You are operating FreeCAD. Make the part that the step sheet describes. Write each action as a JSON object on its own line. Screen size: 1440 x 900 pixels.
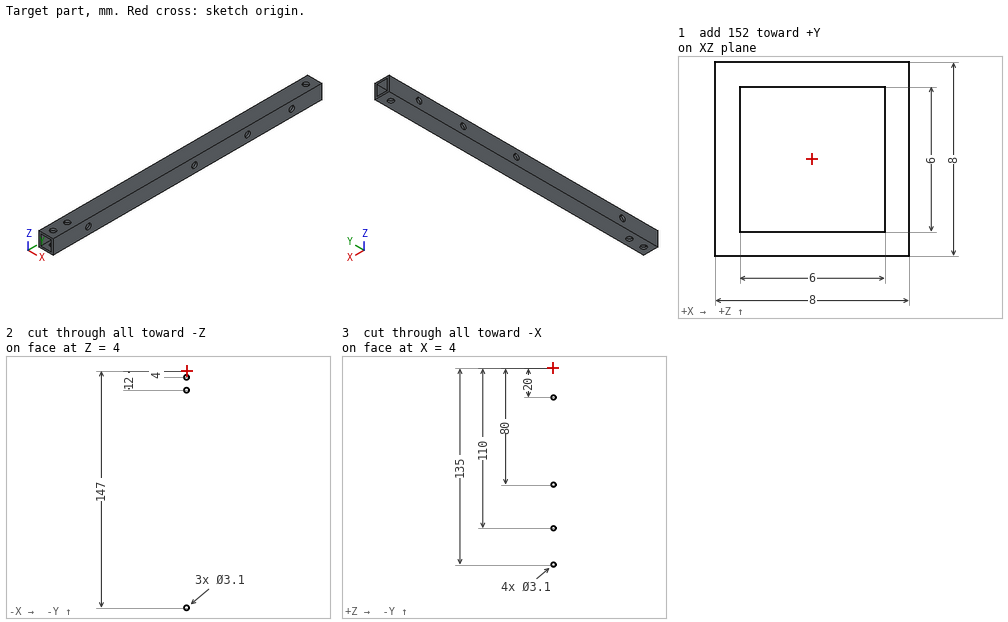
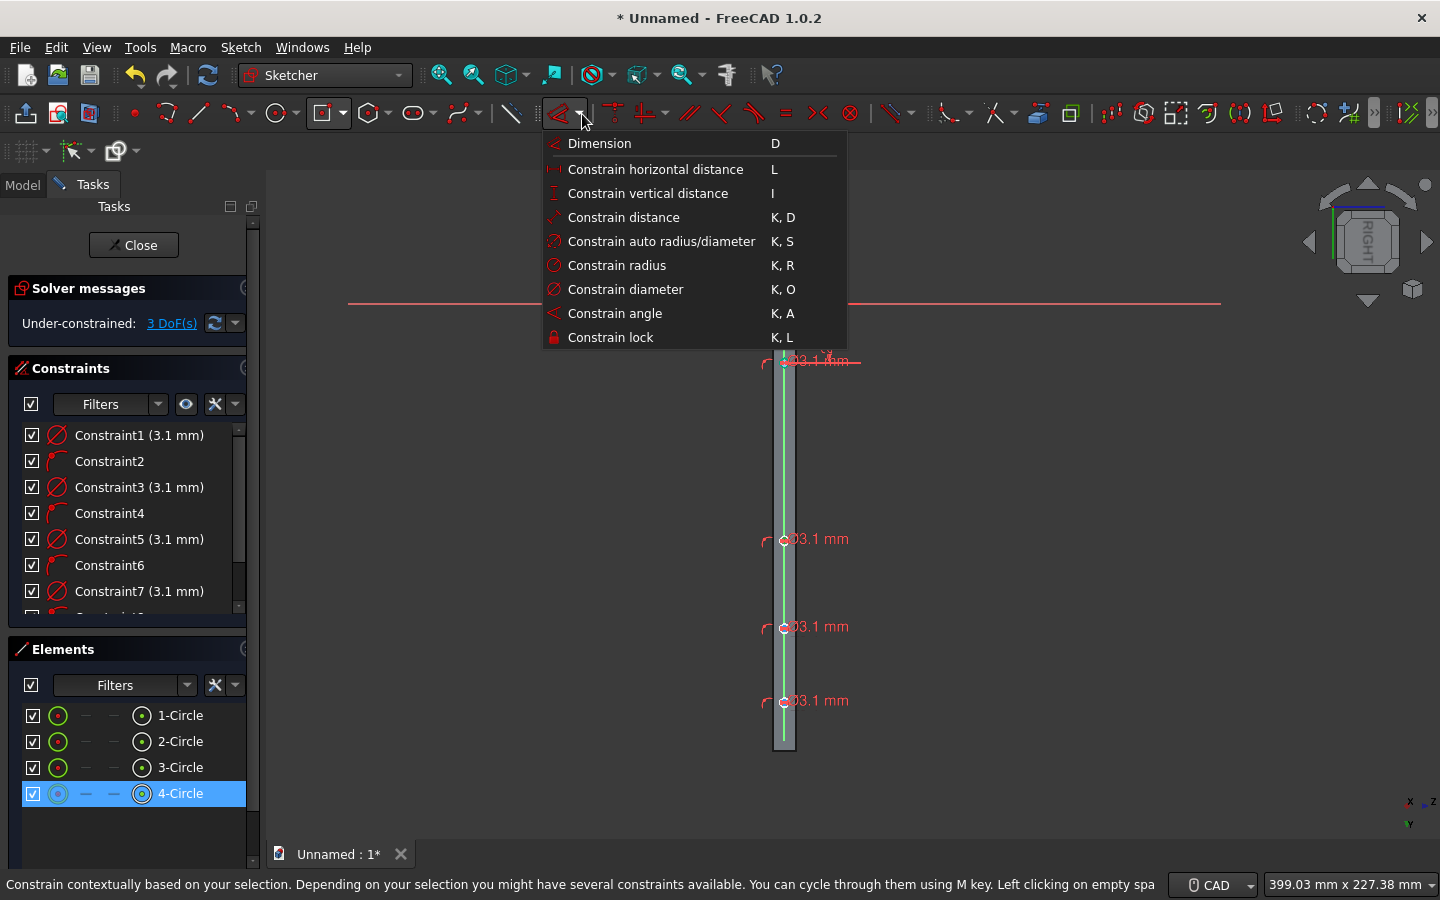
{"action": "left_click", "coordinate": [695, 193]}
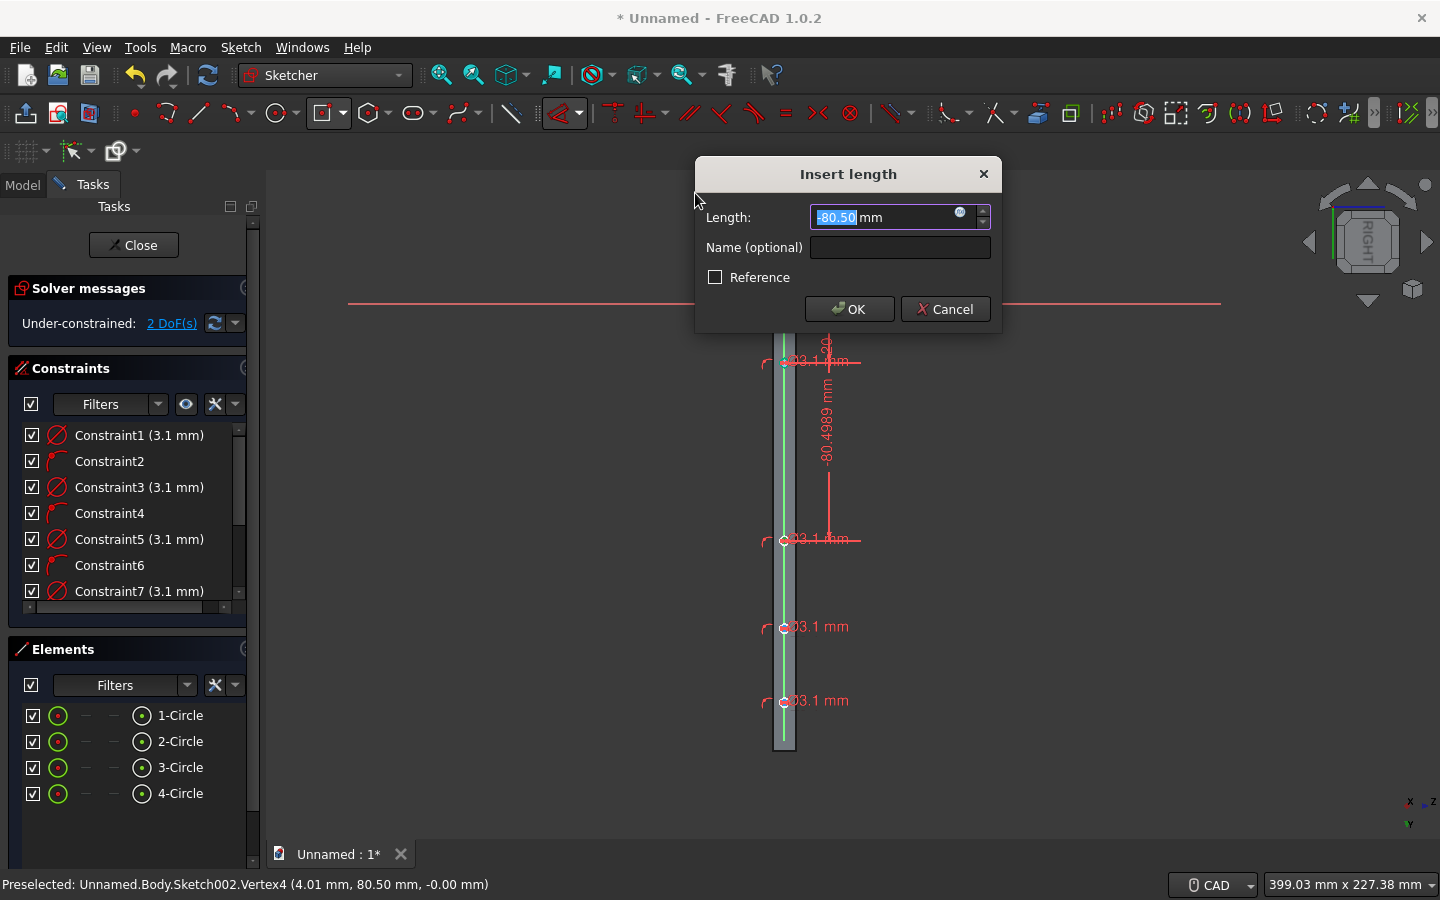
{"action": "type", "text": "-80"}
{"action": "key", "text": "Return"}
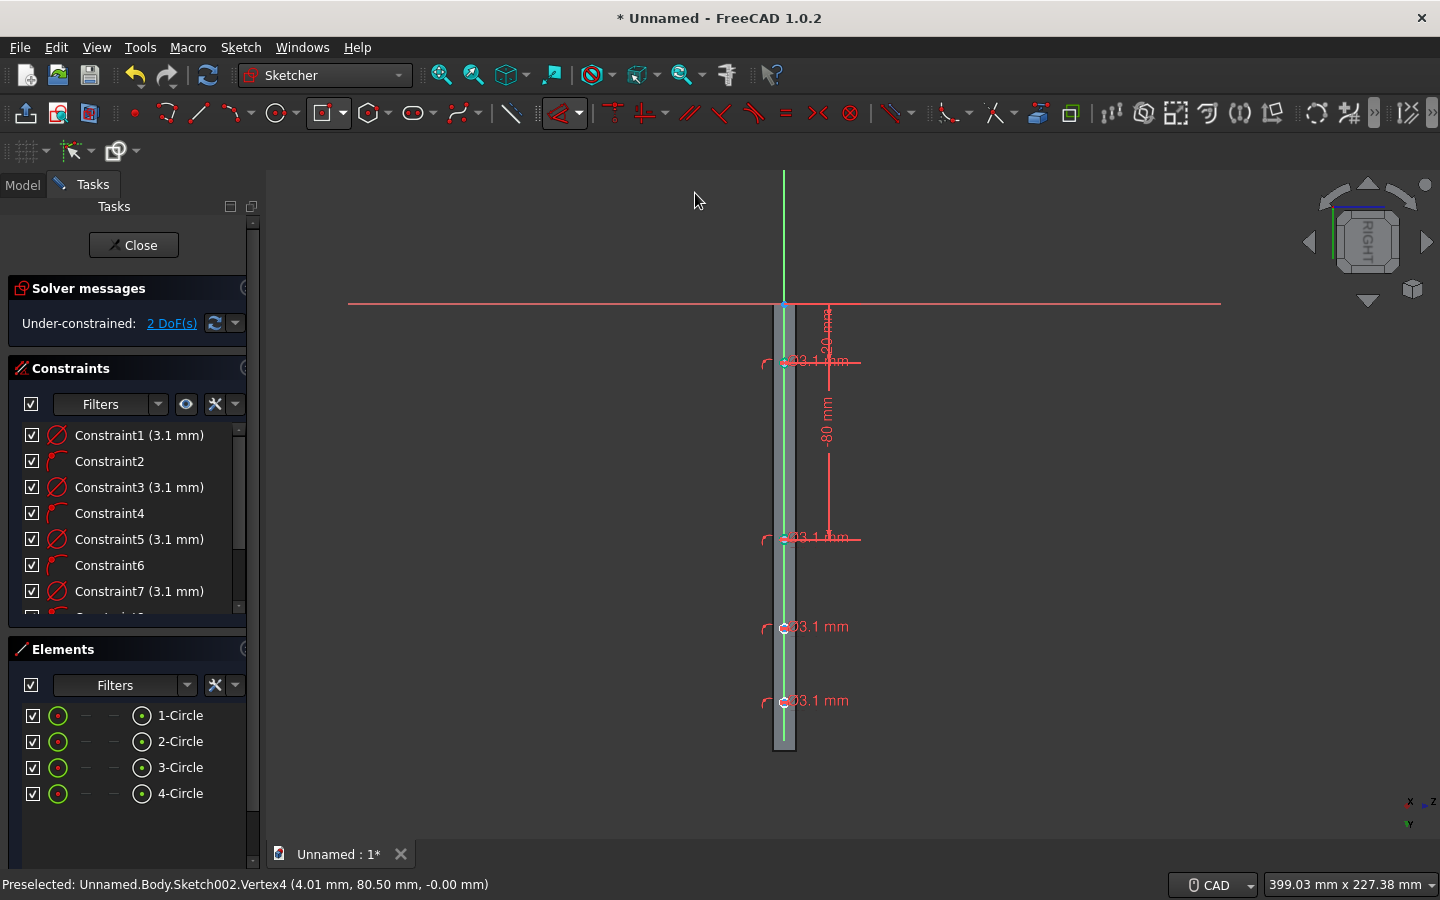
{"action": "left_click", "coordinate": [784, 703]}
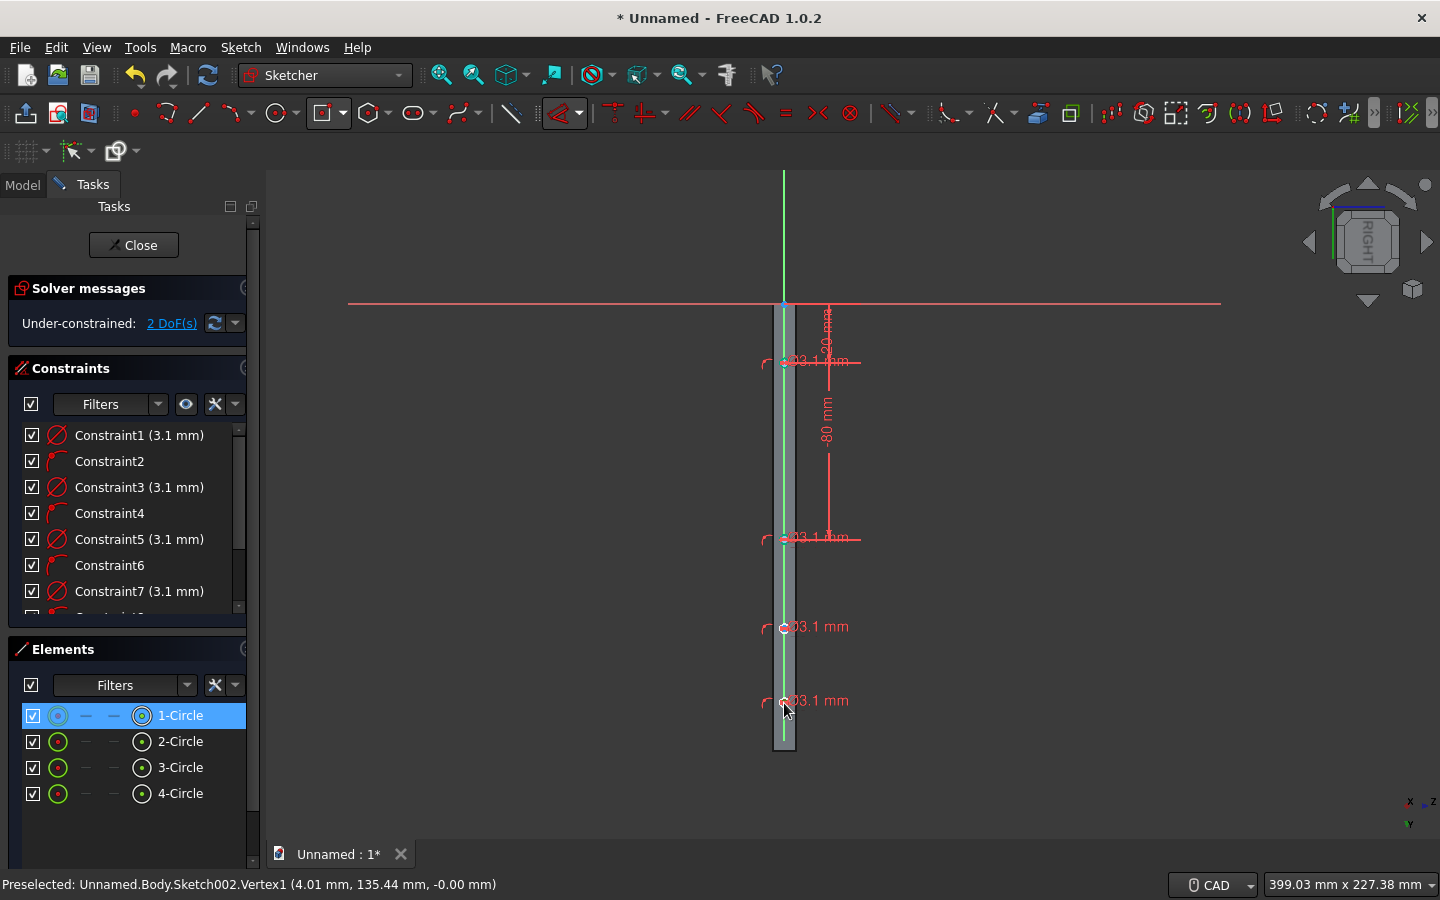
{"action": "key", "text": "i"}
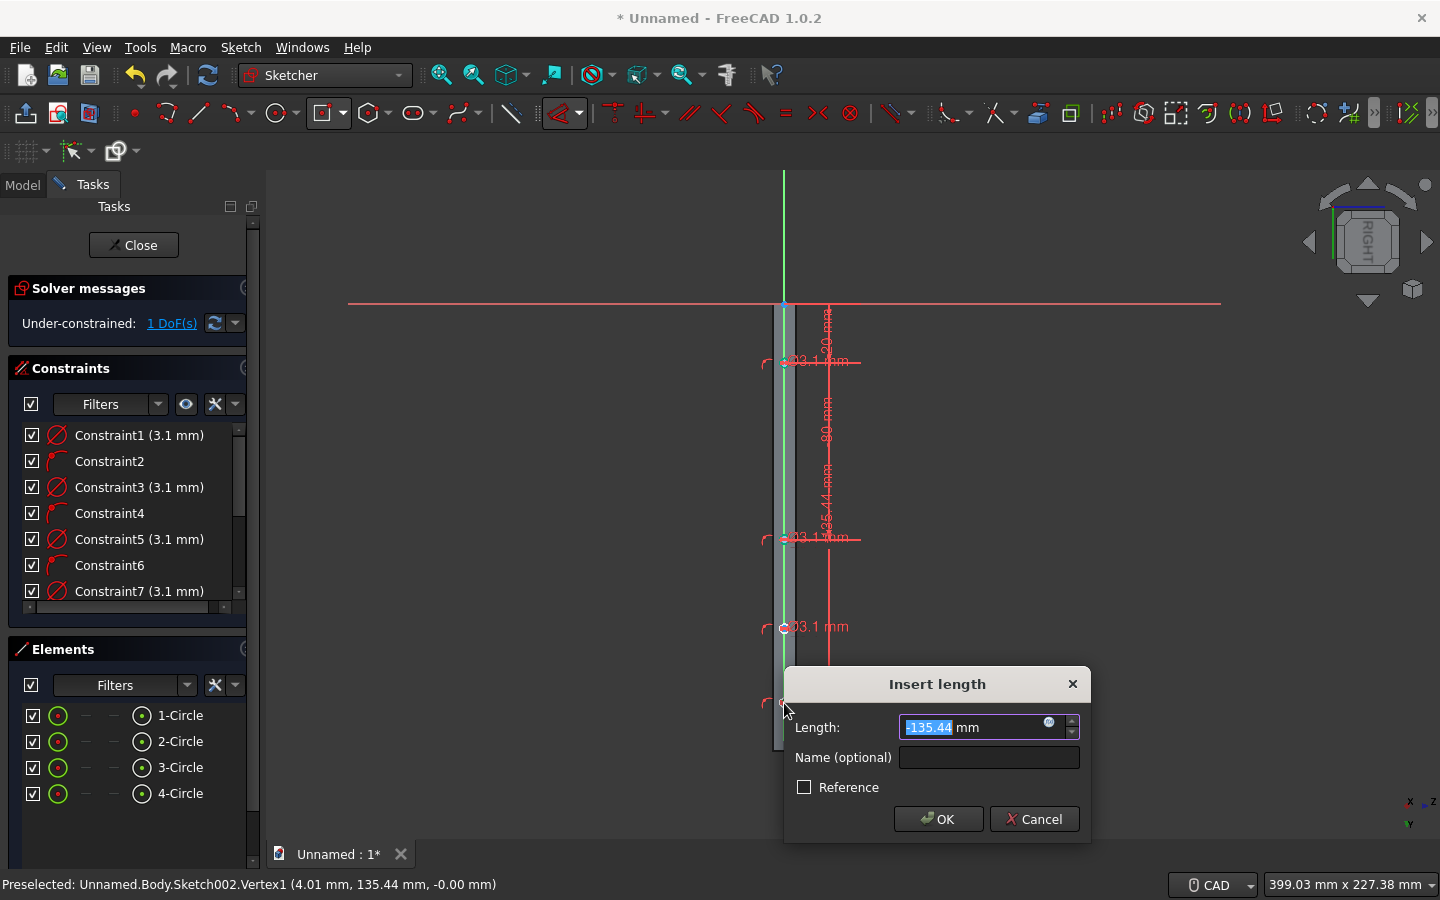
{"action": "type", "text": "-135"}
{"action": "key", "text": "Return"}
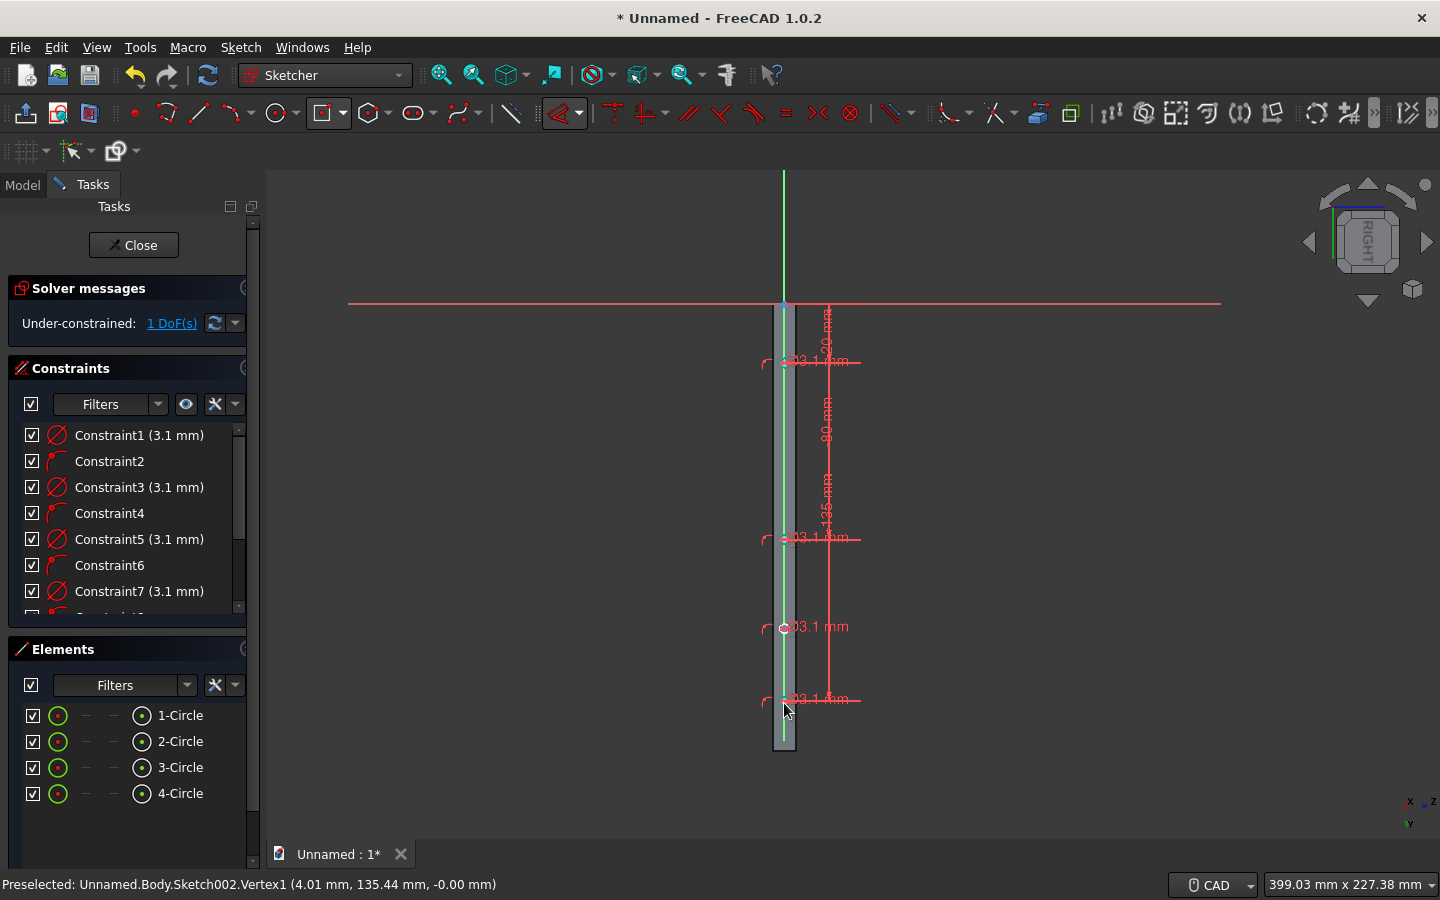
{"action": "left_click", "coordinate": [784, 629]}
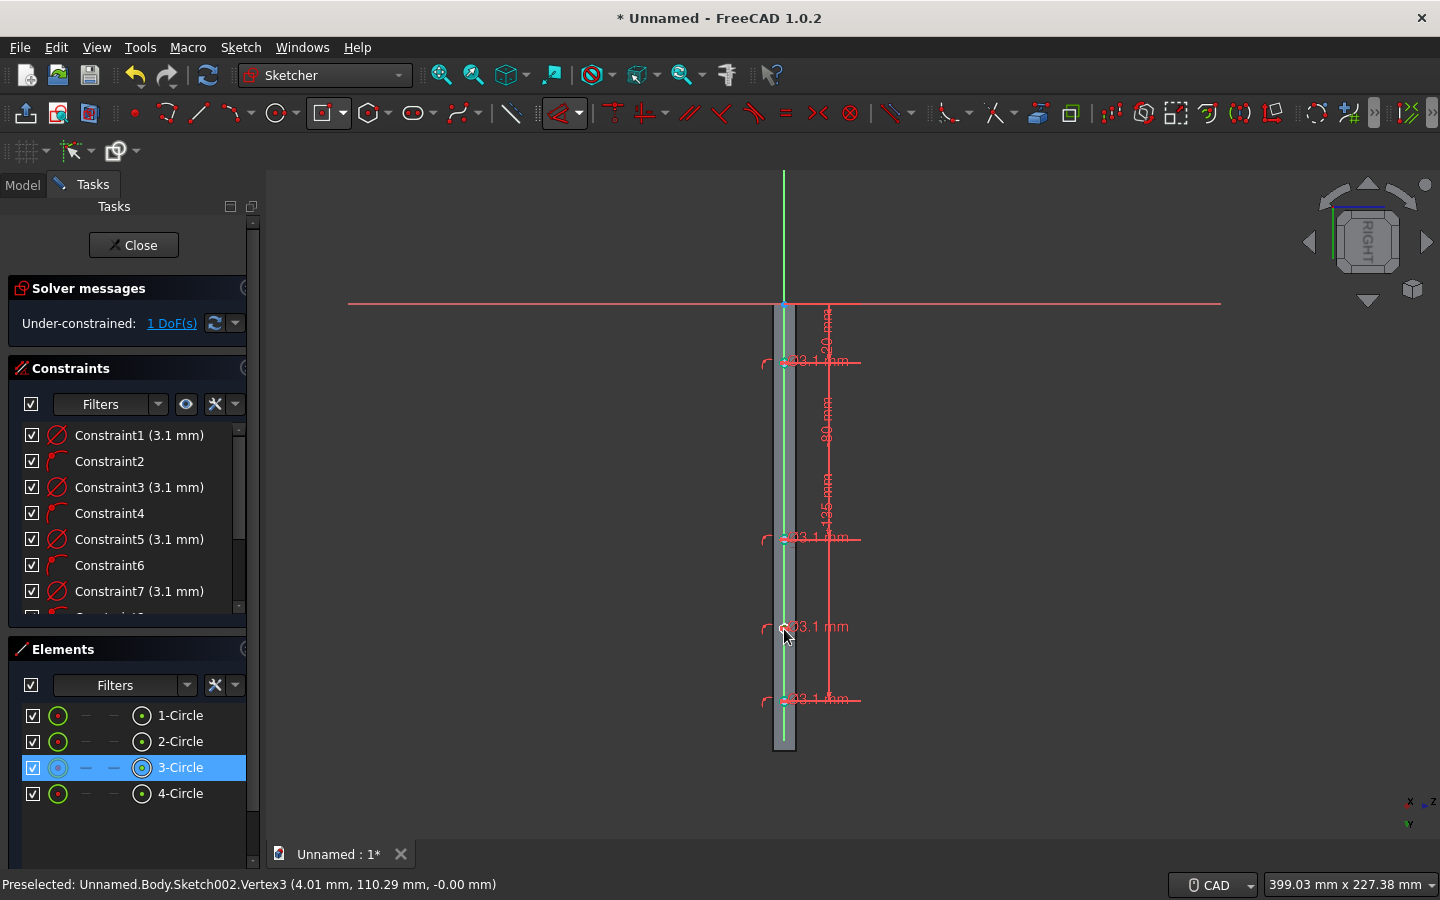
{"action": "left_click", "coordinate": [582, 114]}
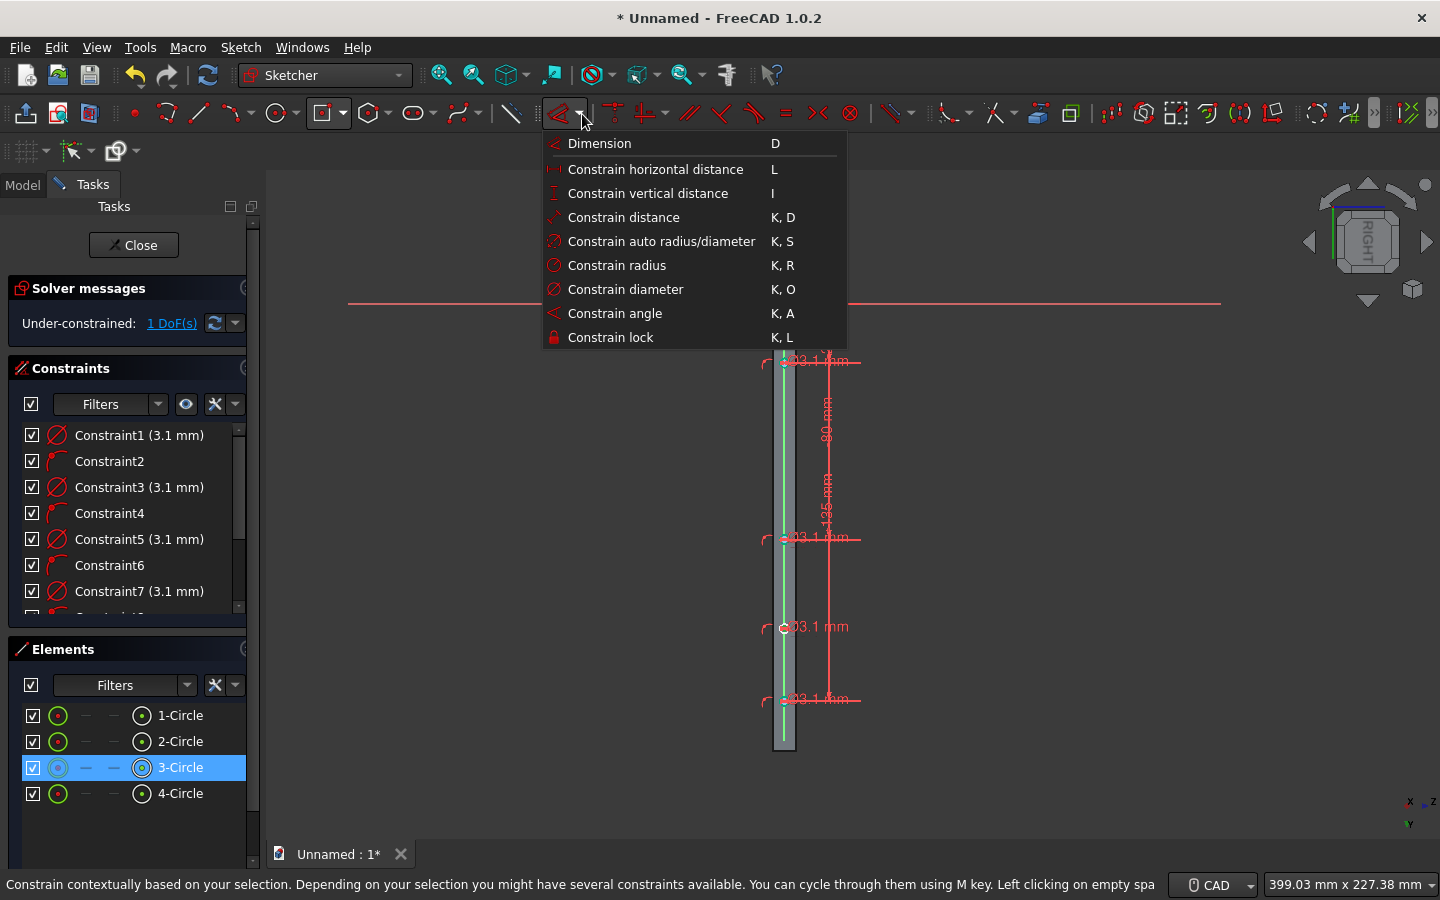
{"action": "left_click", "coordinate": [695, 193]}